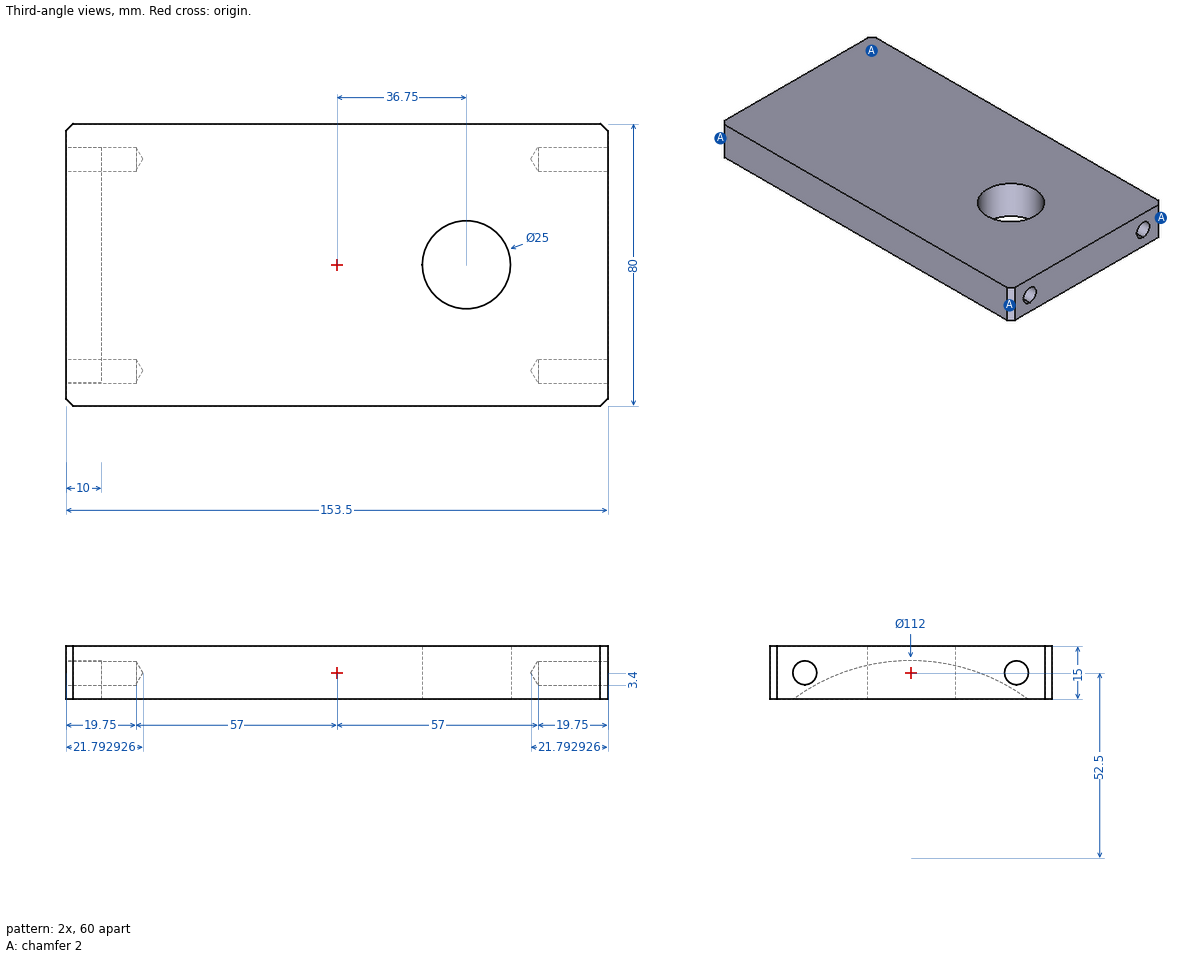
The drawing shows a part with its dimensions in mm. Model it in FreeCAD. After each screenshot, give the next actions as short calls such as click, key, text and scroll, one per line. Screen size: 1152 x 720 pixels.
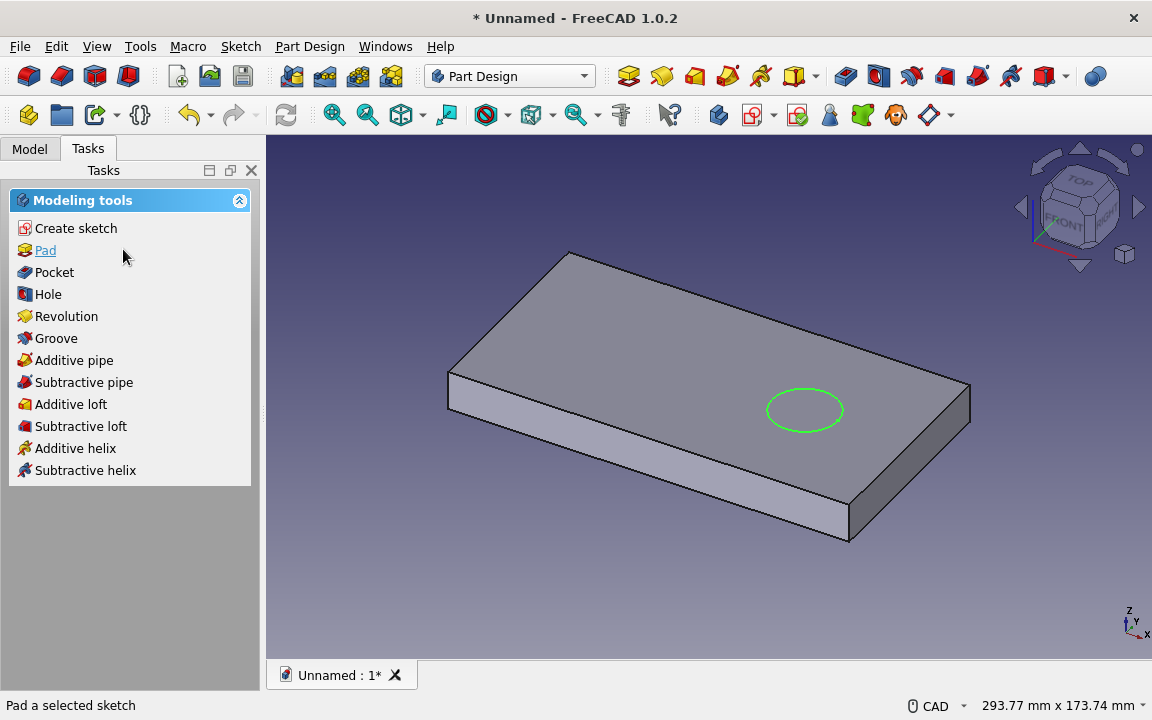
click(846, 76)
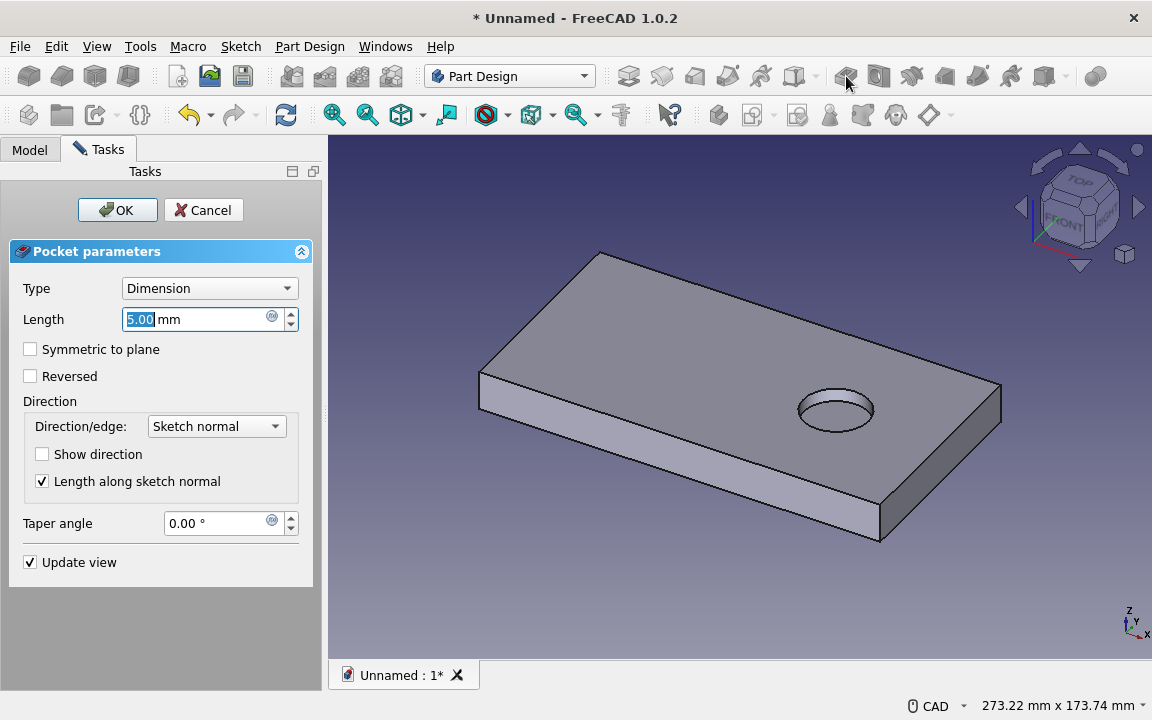
click(210, 288)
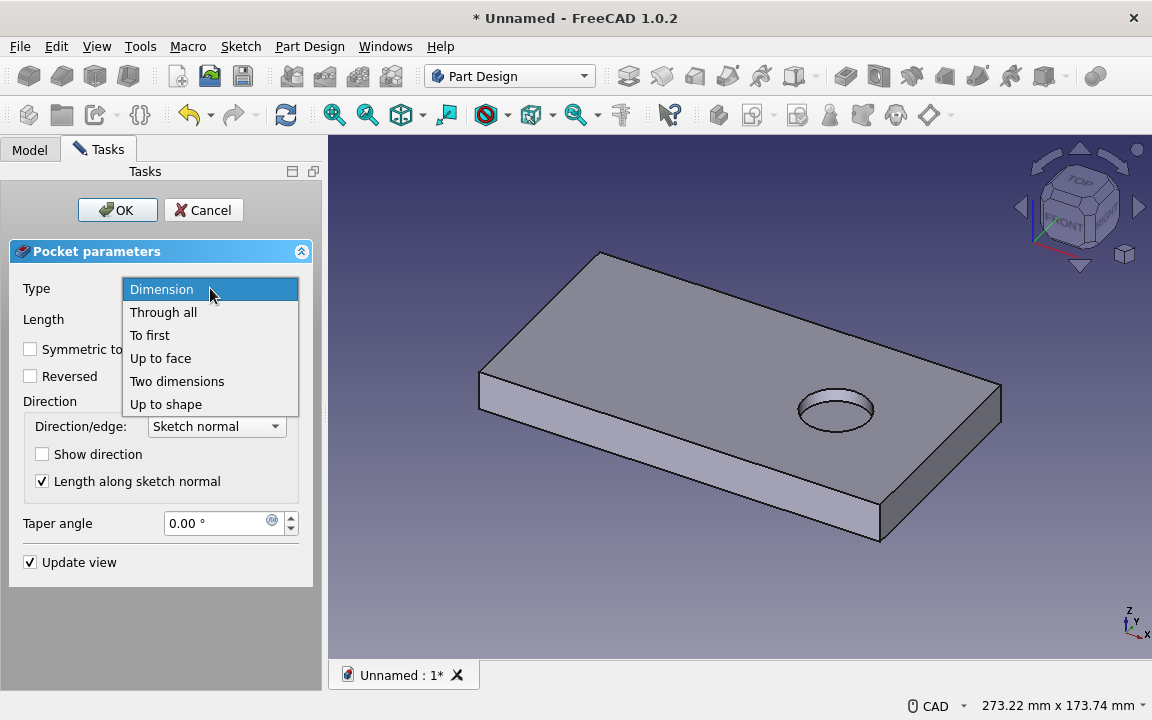
click(208, 312)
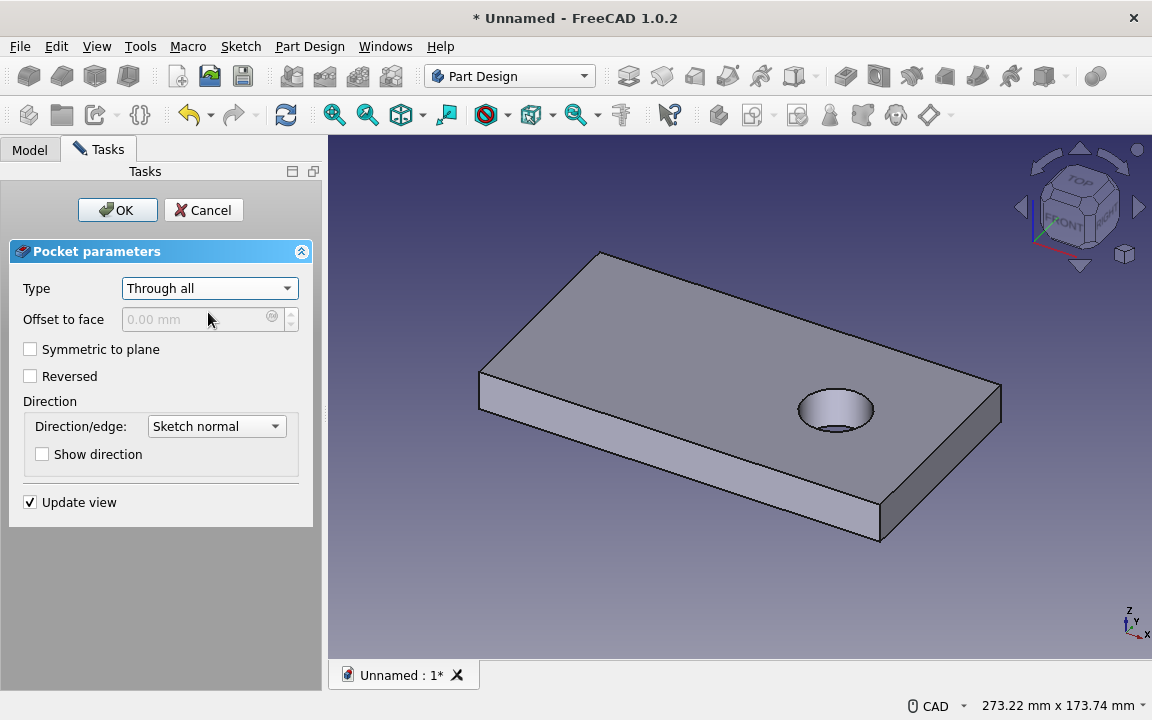
click(118, 210)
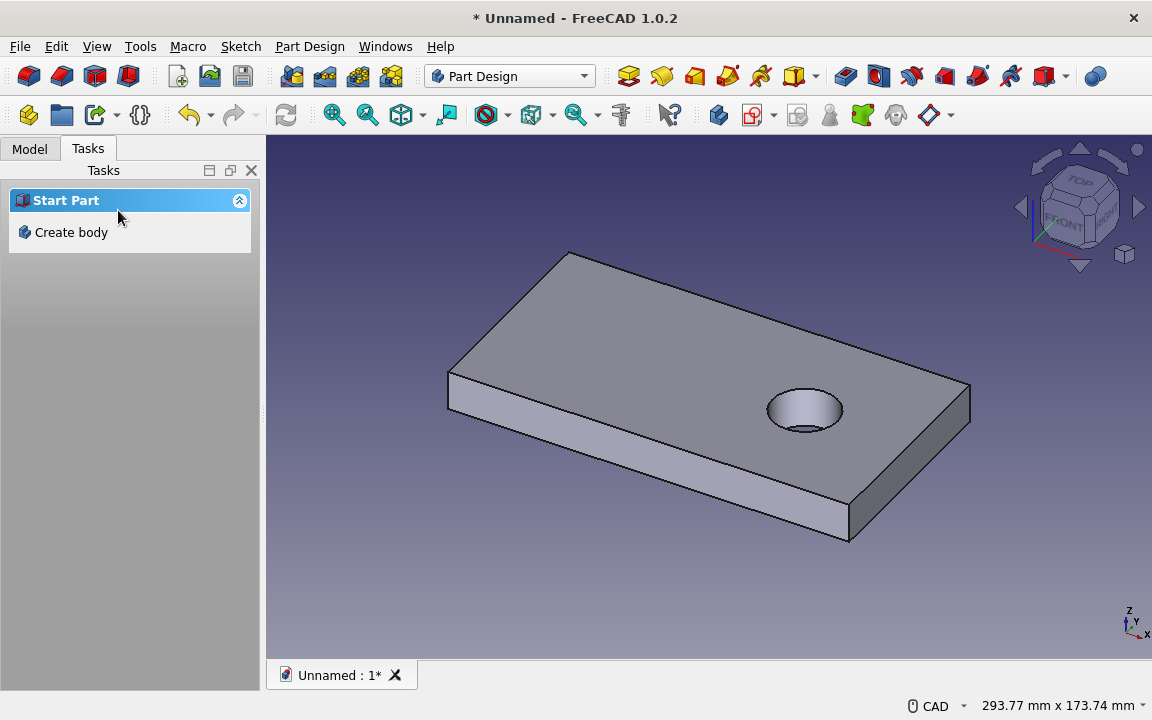
click(30, 148)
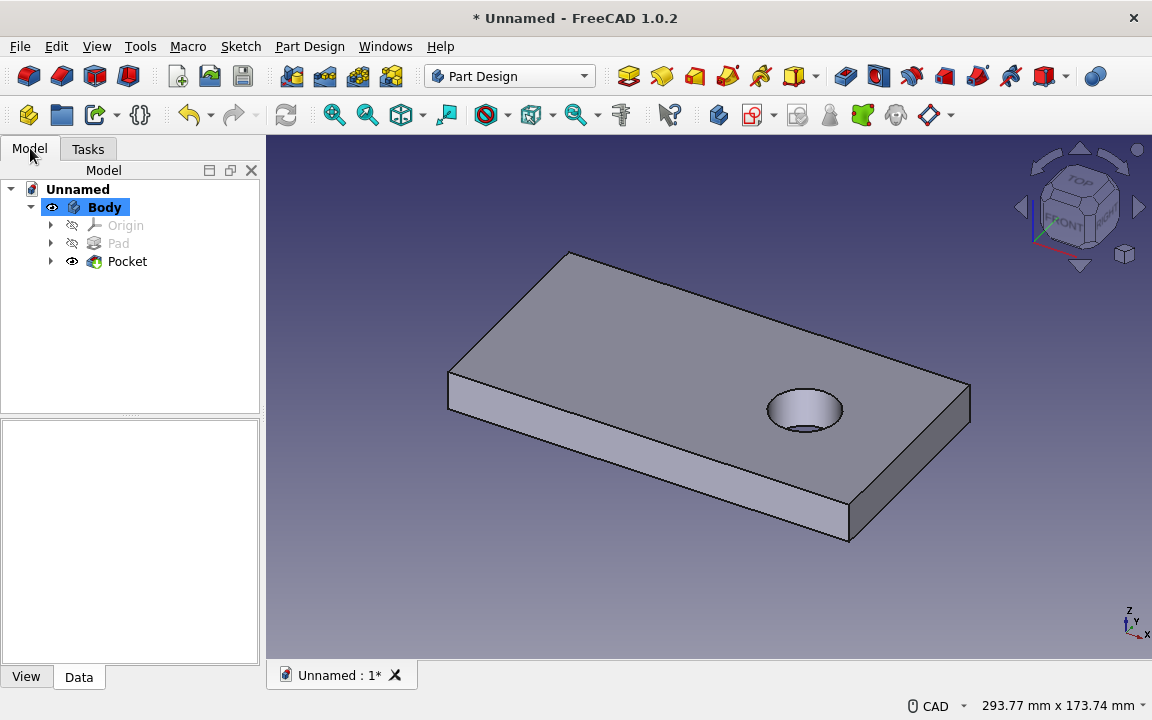
click(51, 225)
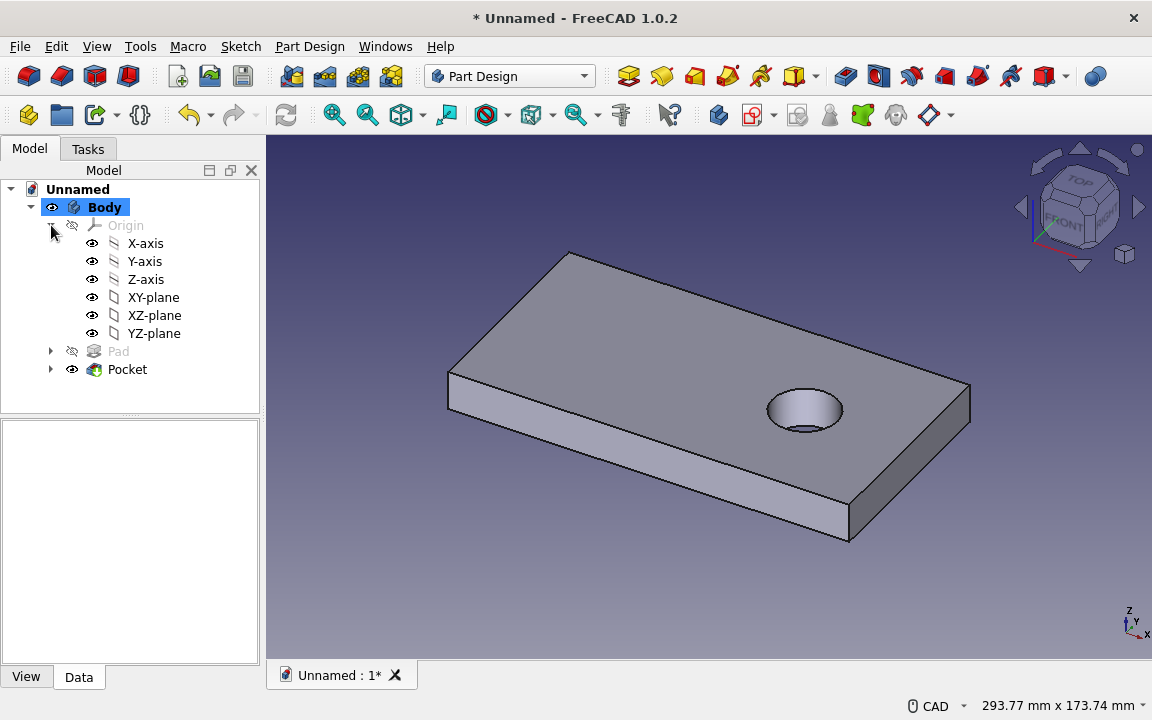
click(137, 315)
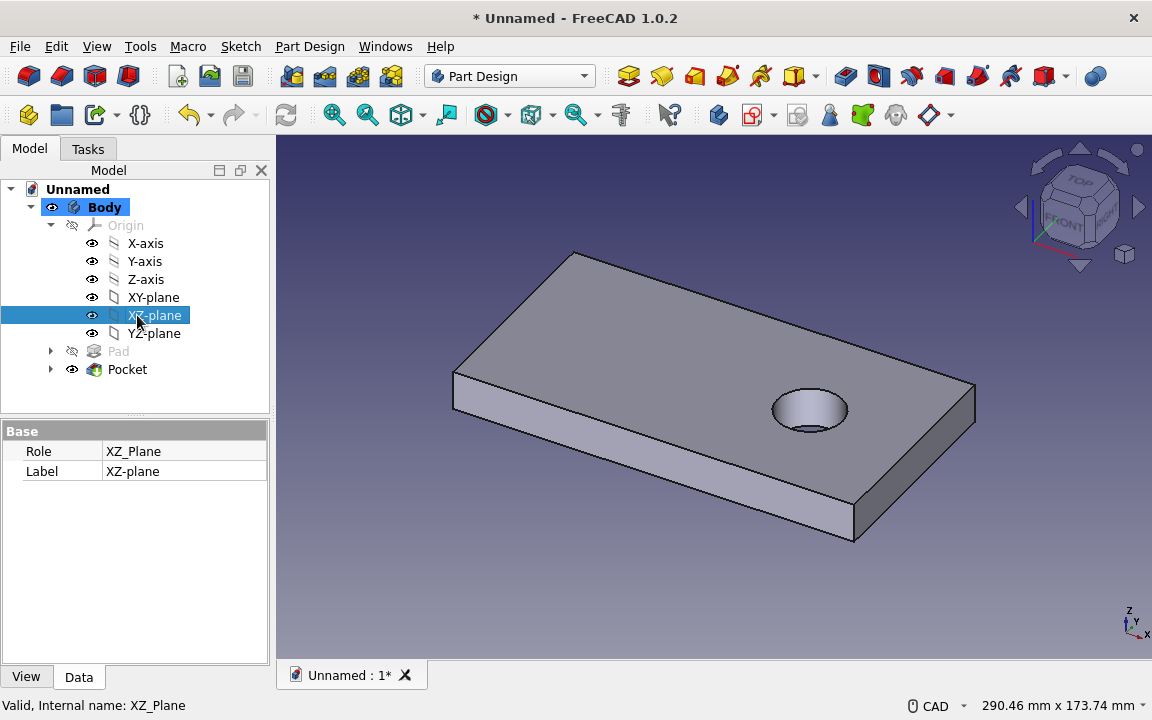
click(928, 116)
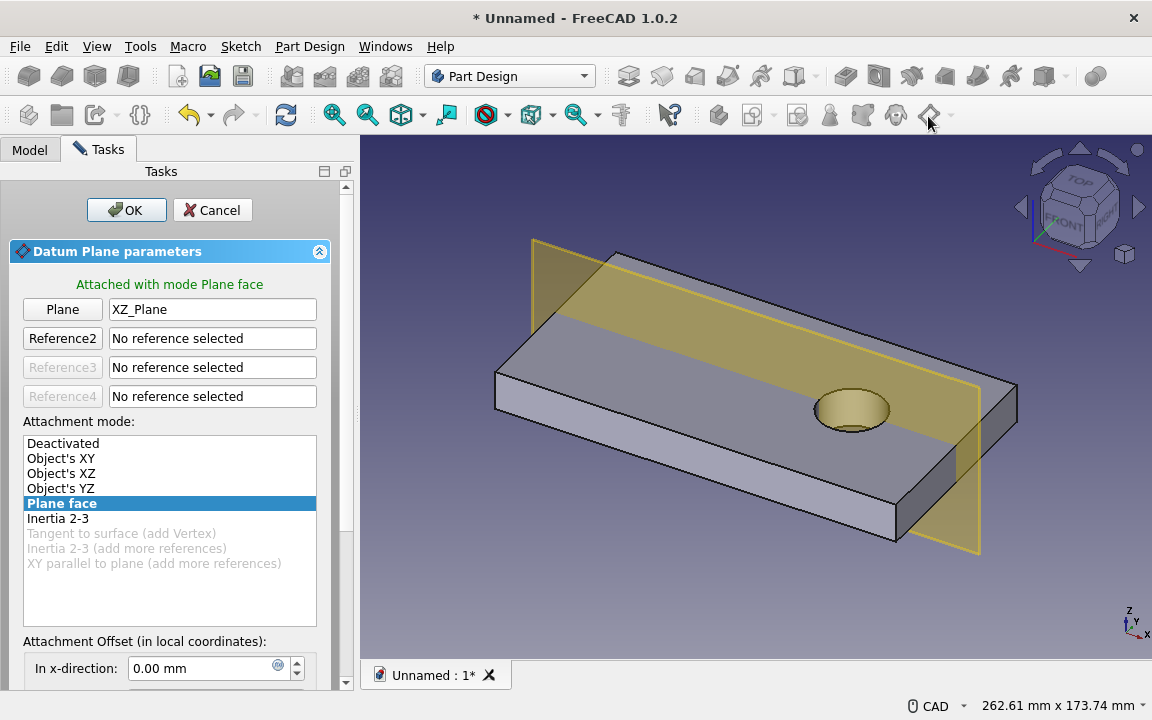
scroll(346, 436, down, 2)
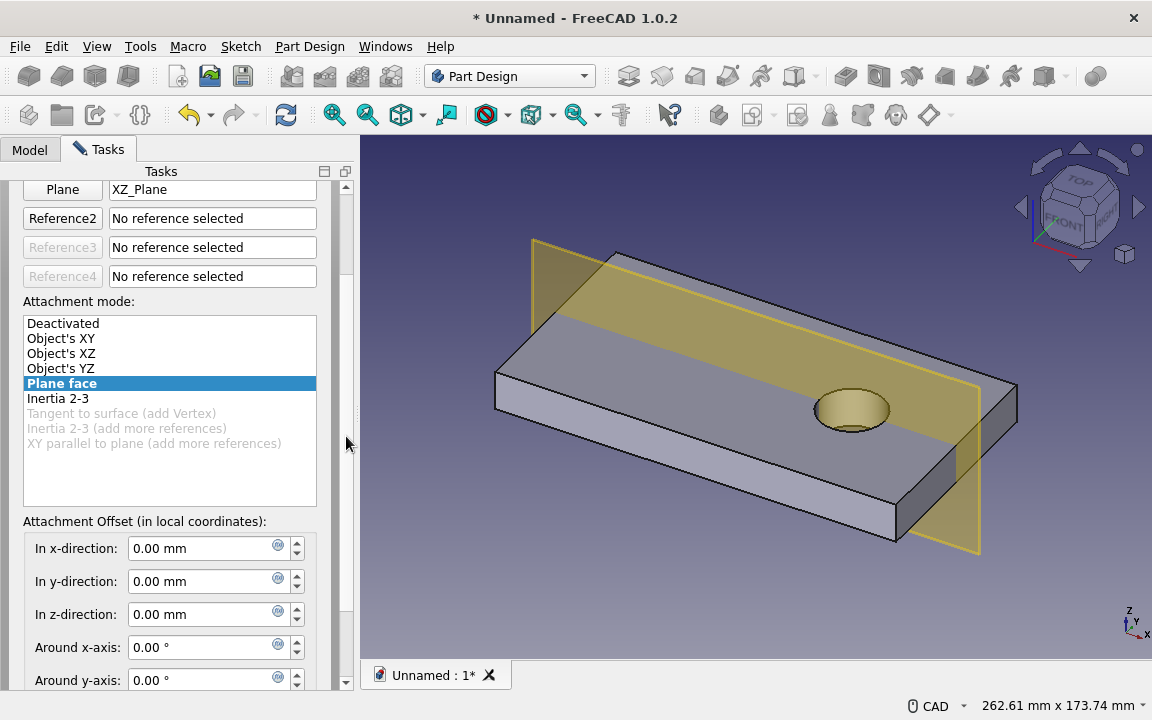
triple_click(210, 614)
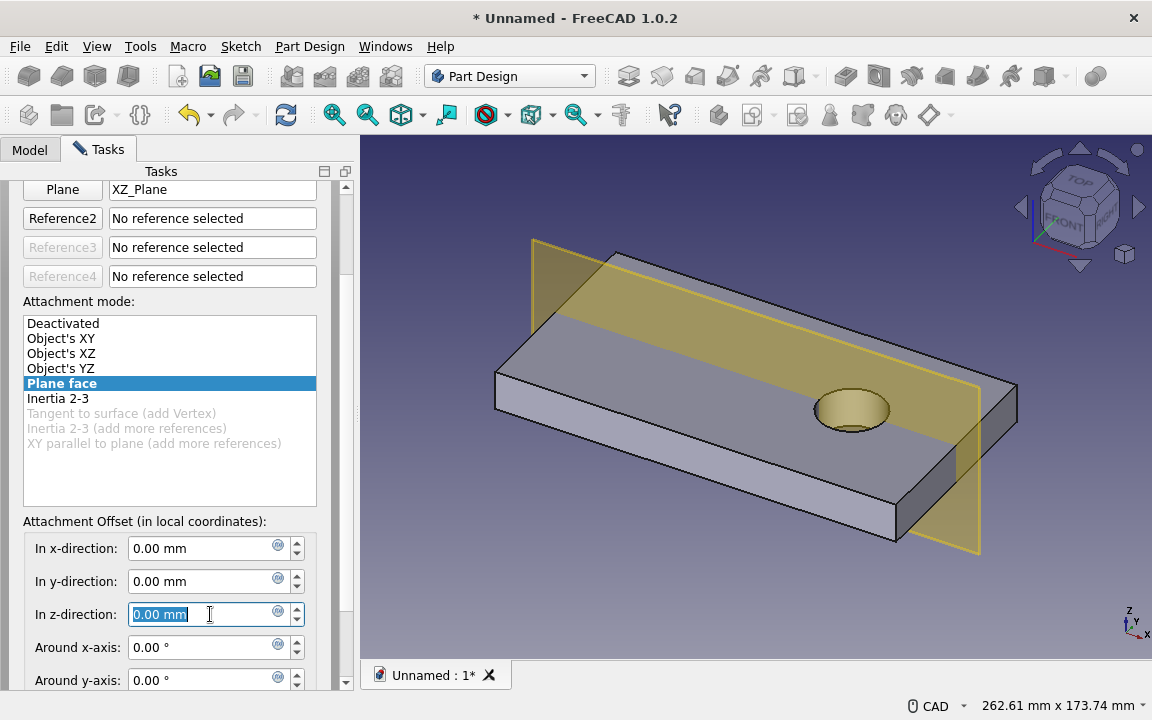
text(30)
key(Tab)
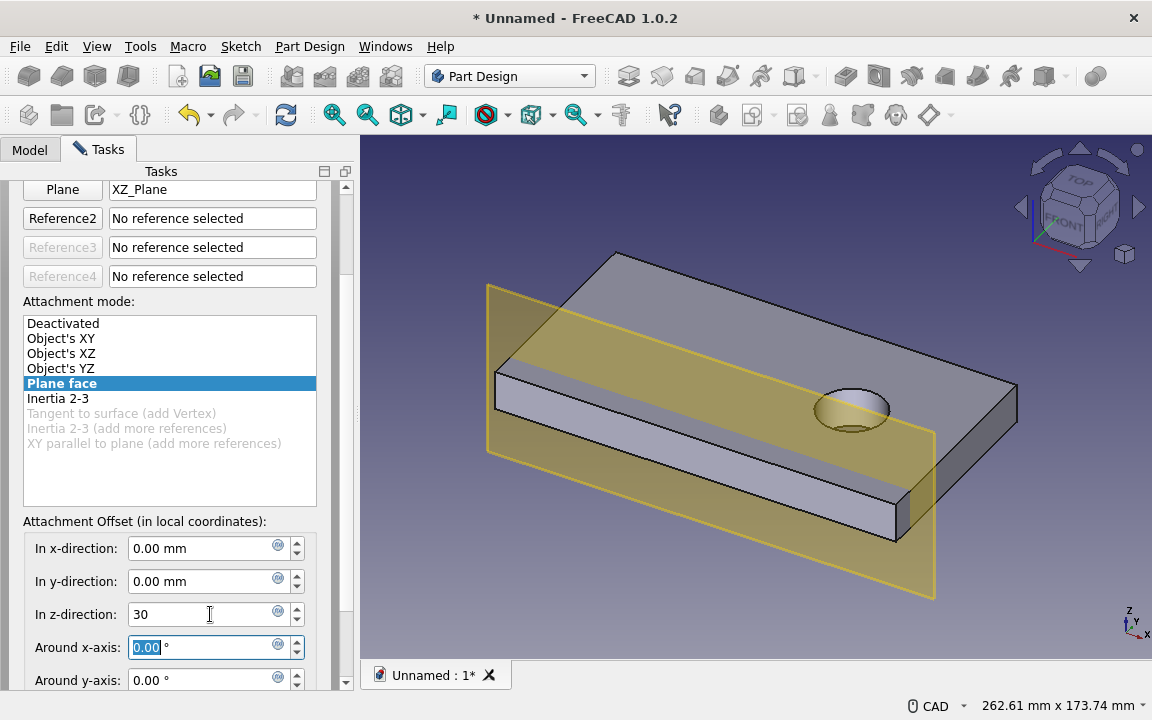
scroll(346, 436, up, 3)